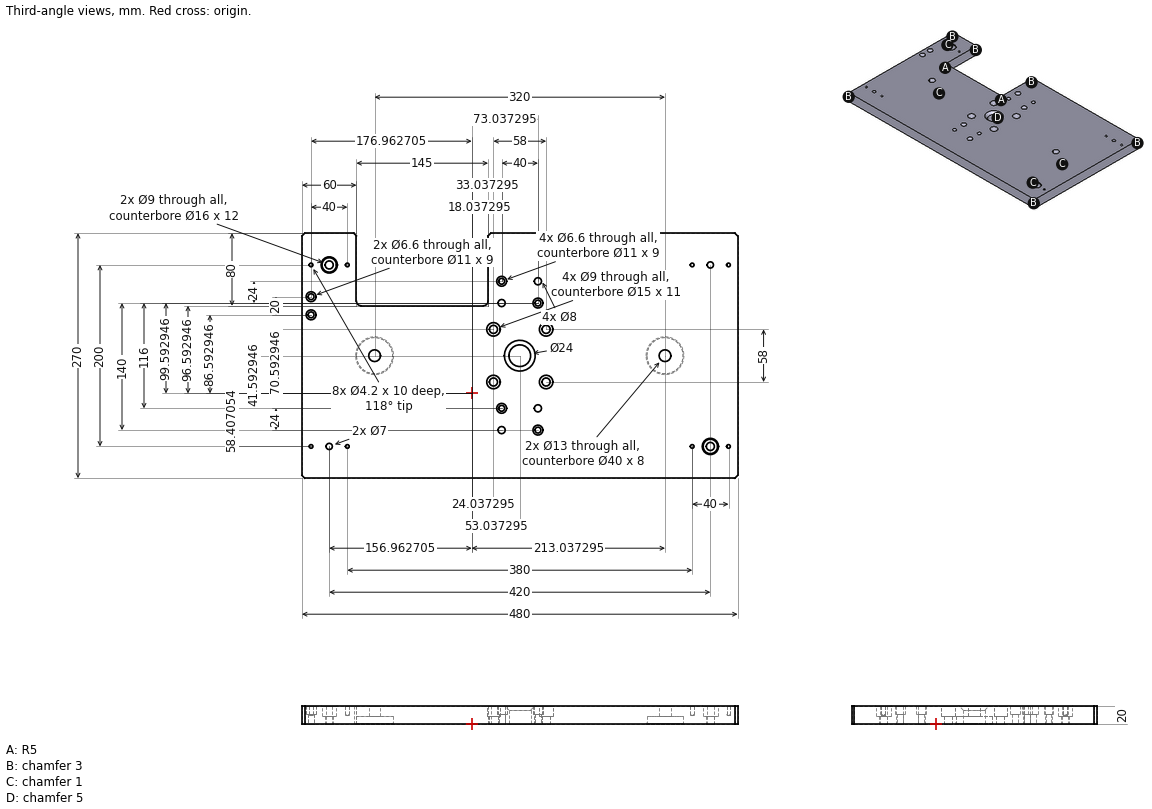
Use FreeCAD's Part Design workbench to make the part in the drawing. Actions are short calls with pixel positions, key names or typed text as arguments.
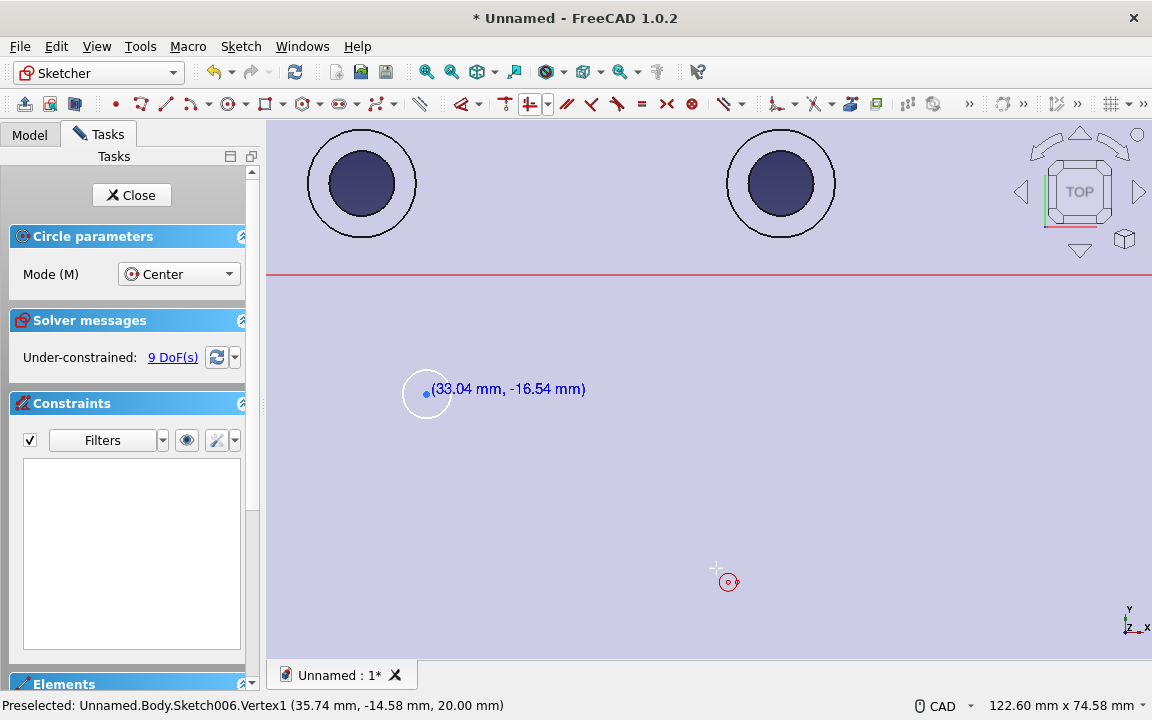
click(716, 567)
click(733, 550)
key(Escape)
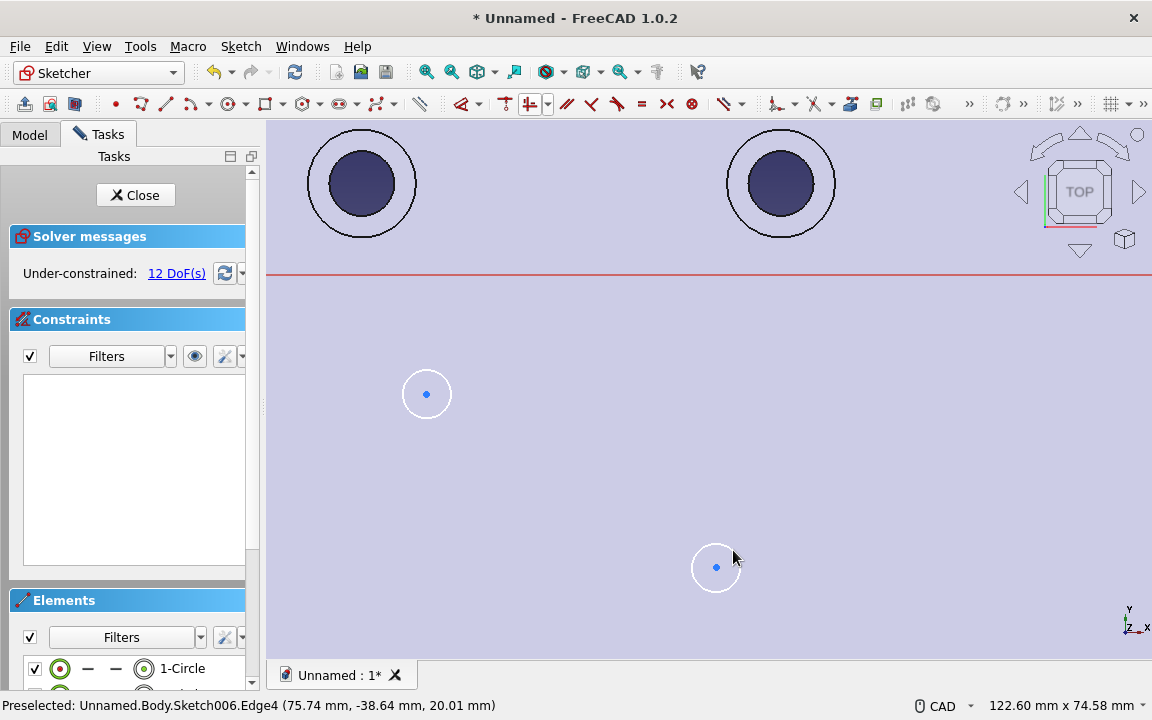
scroll(717, 569, down, 6)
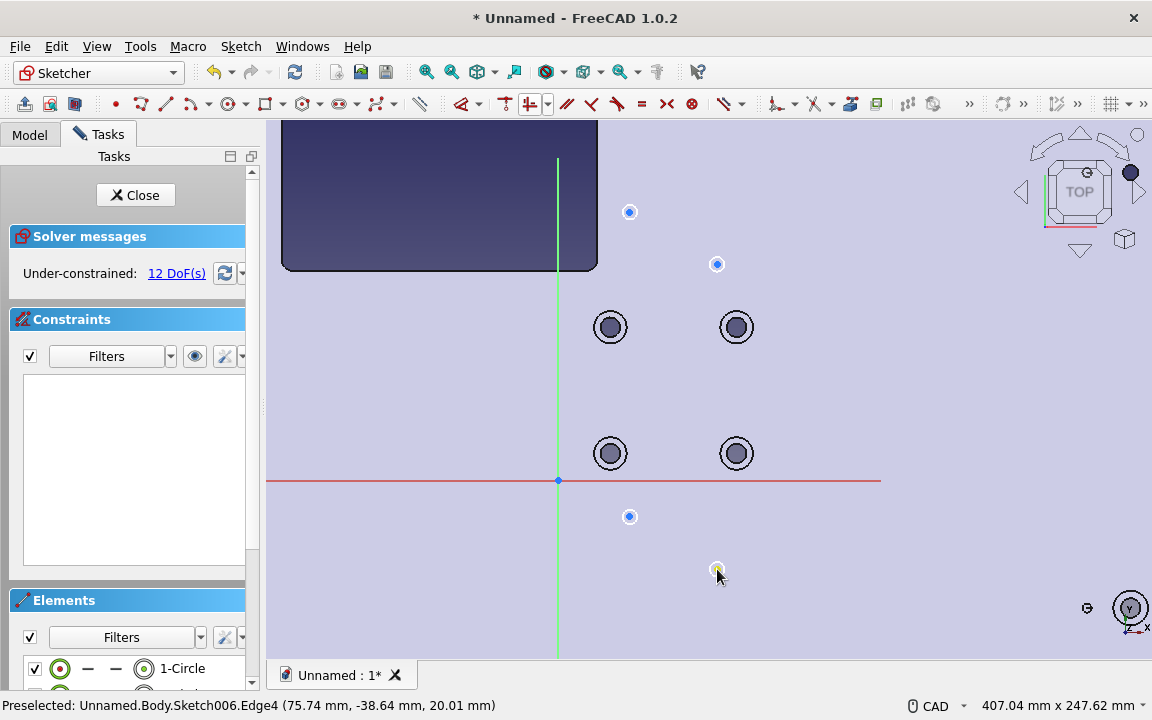
scroll(635, 207, up, 4)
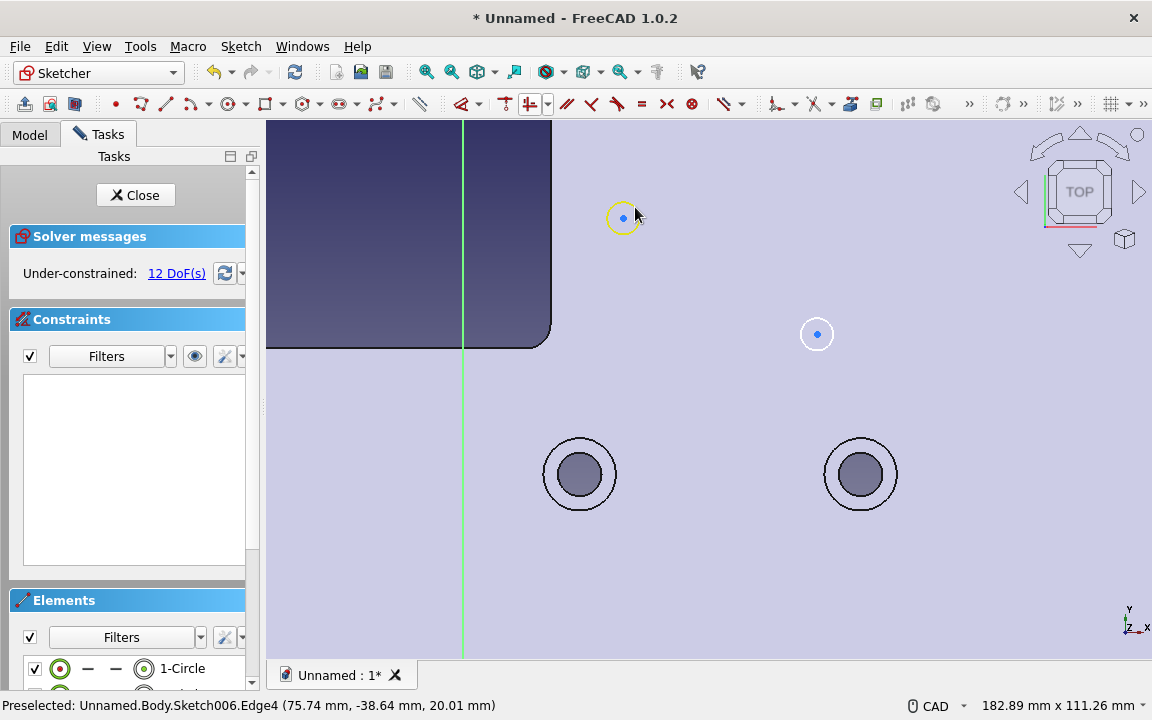
click(635, 207)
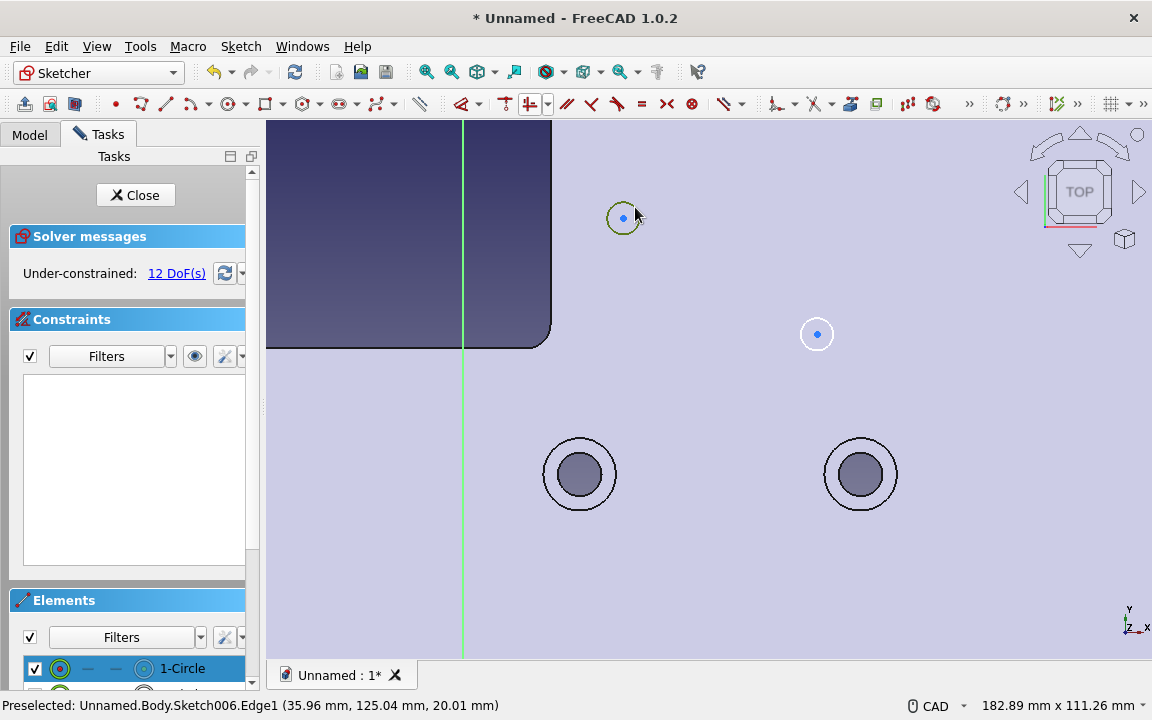
click(828, 323)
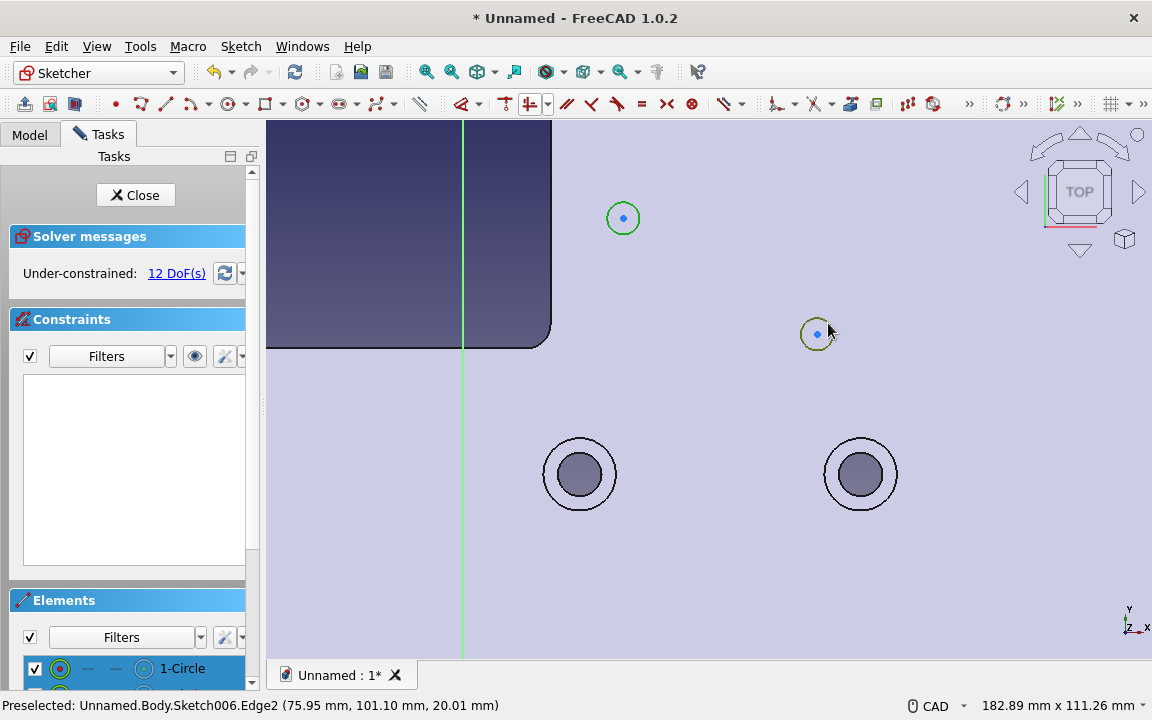
scroll(634, 206, down, 4)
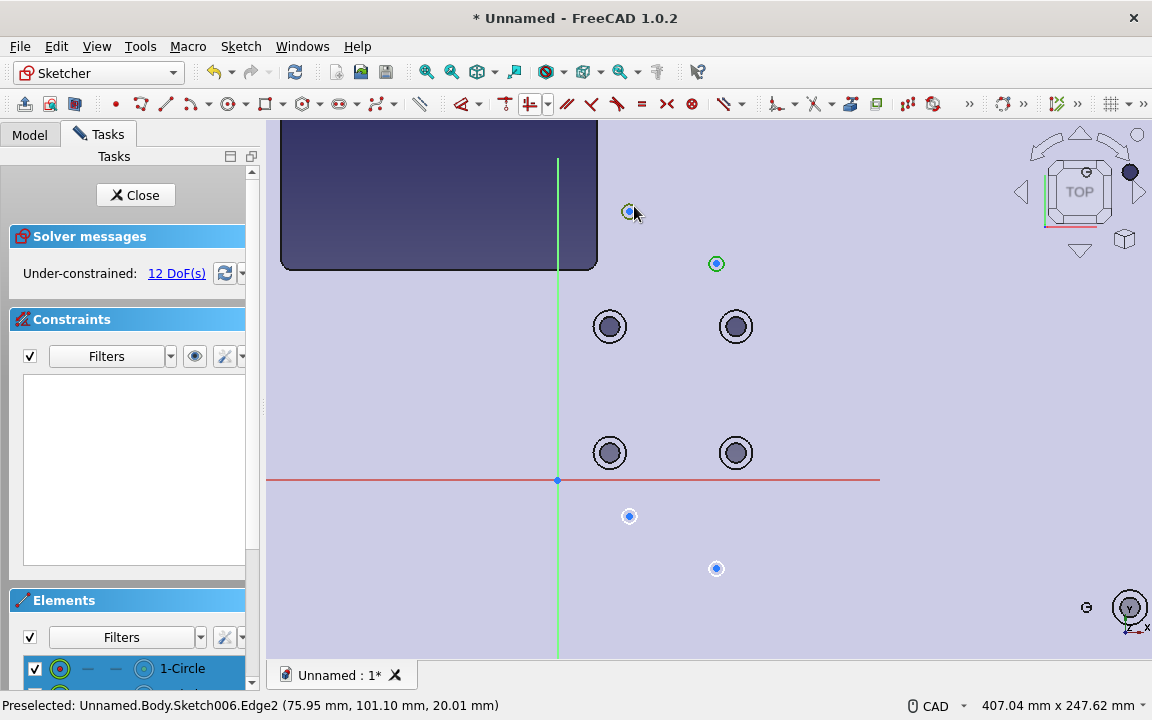
scroll(635, 511, up, 4)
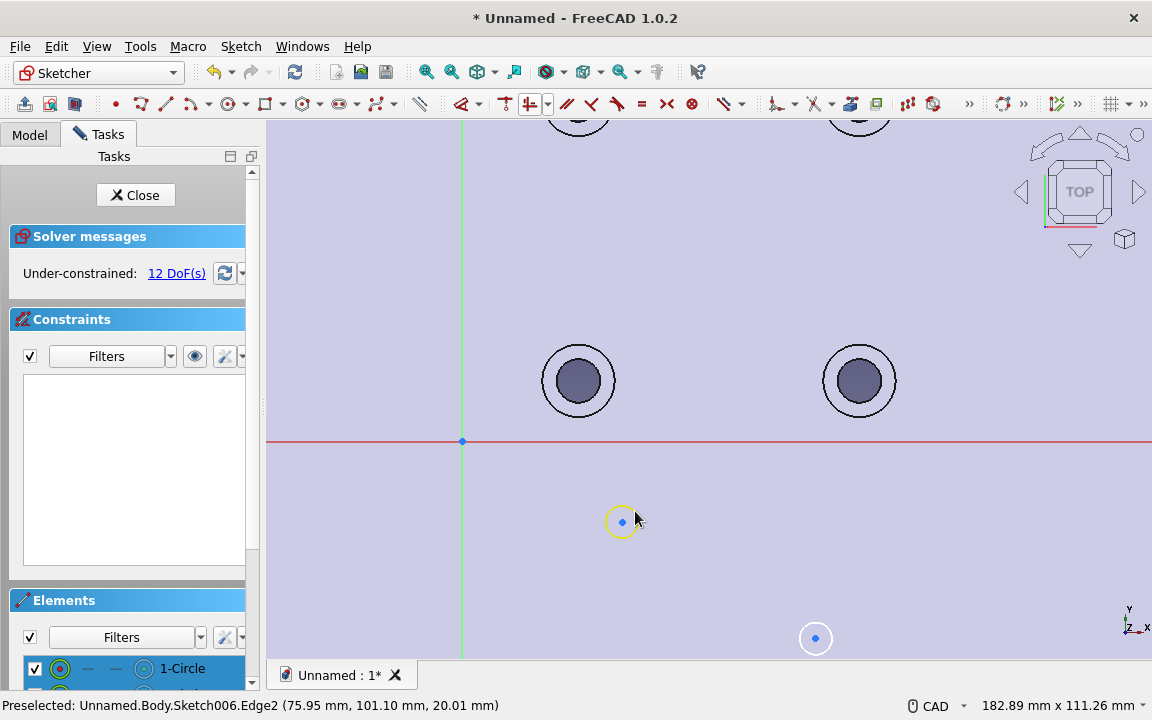
click(633, 511)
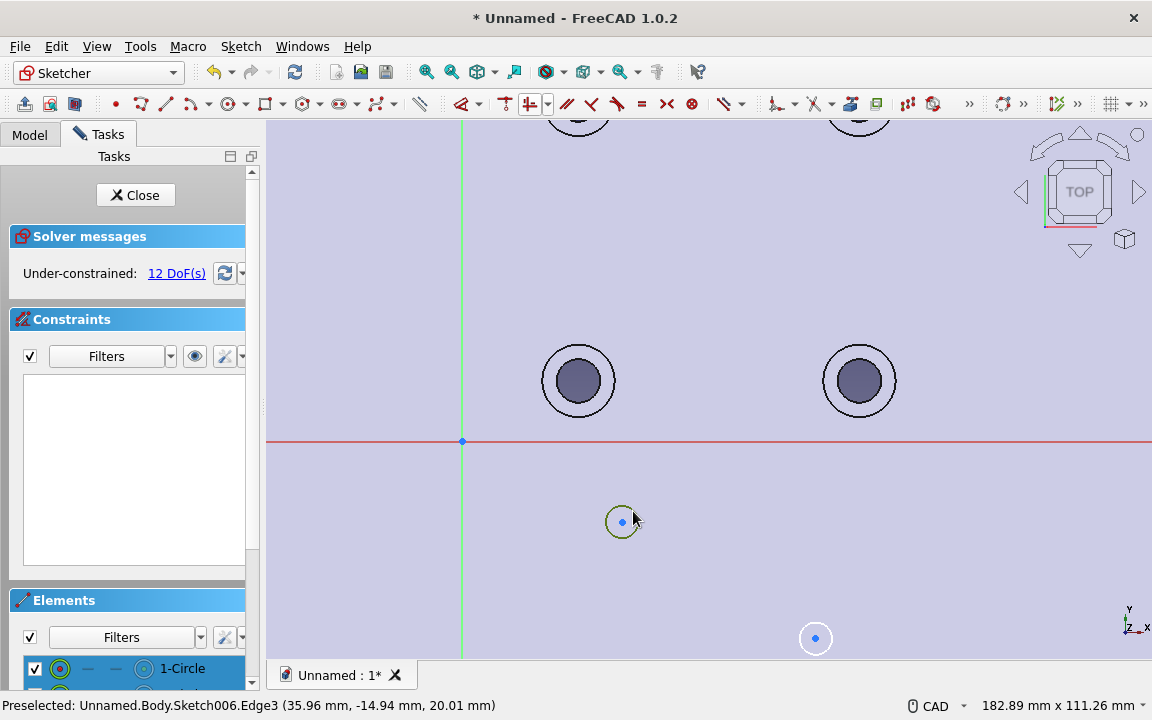
click(827, 627)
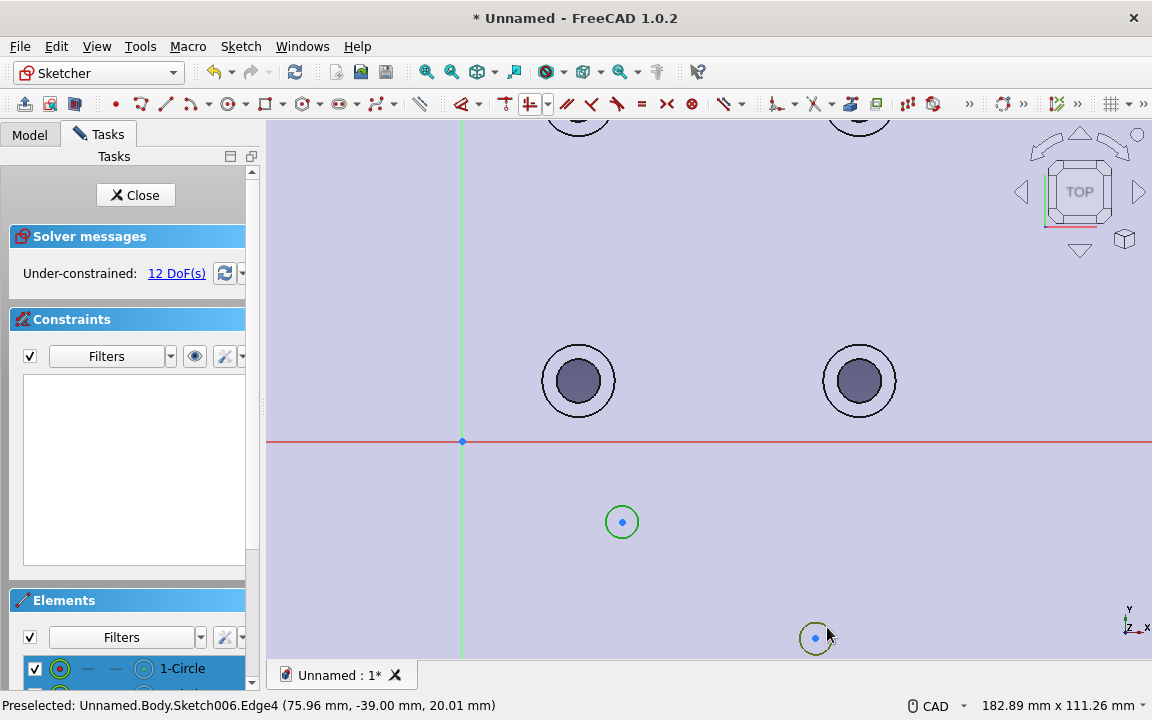
key(e)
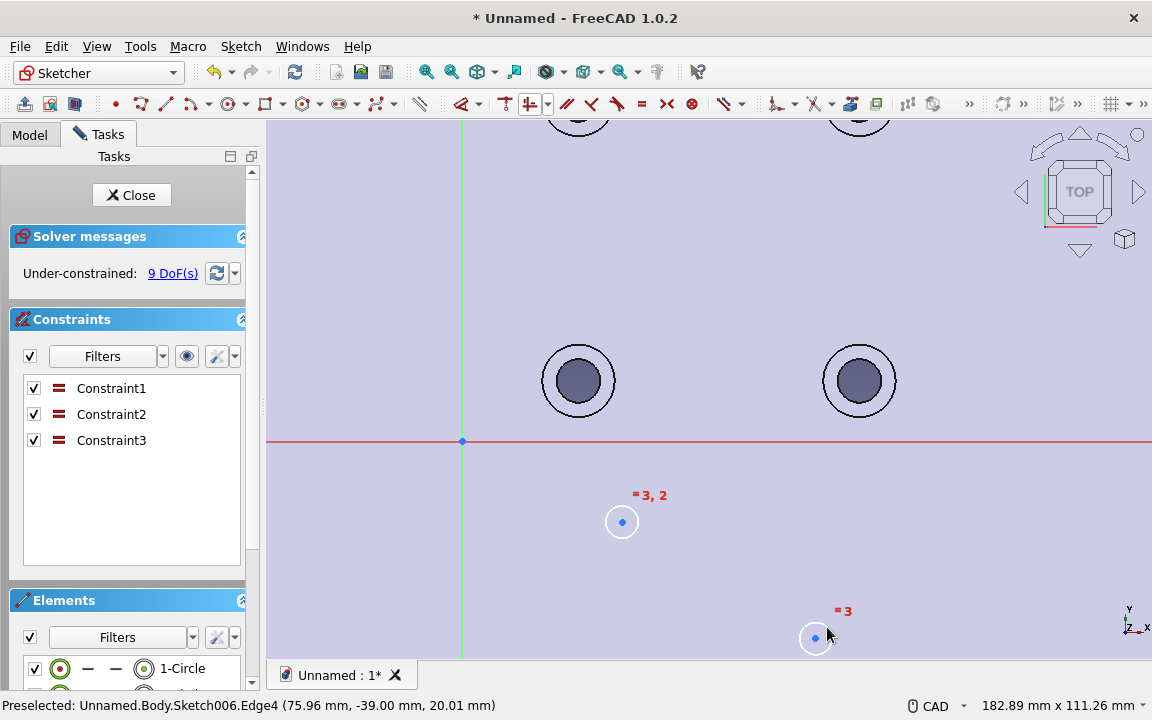
scroll(635, 511, down, 4)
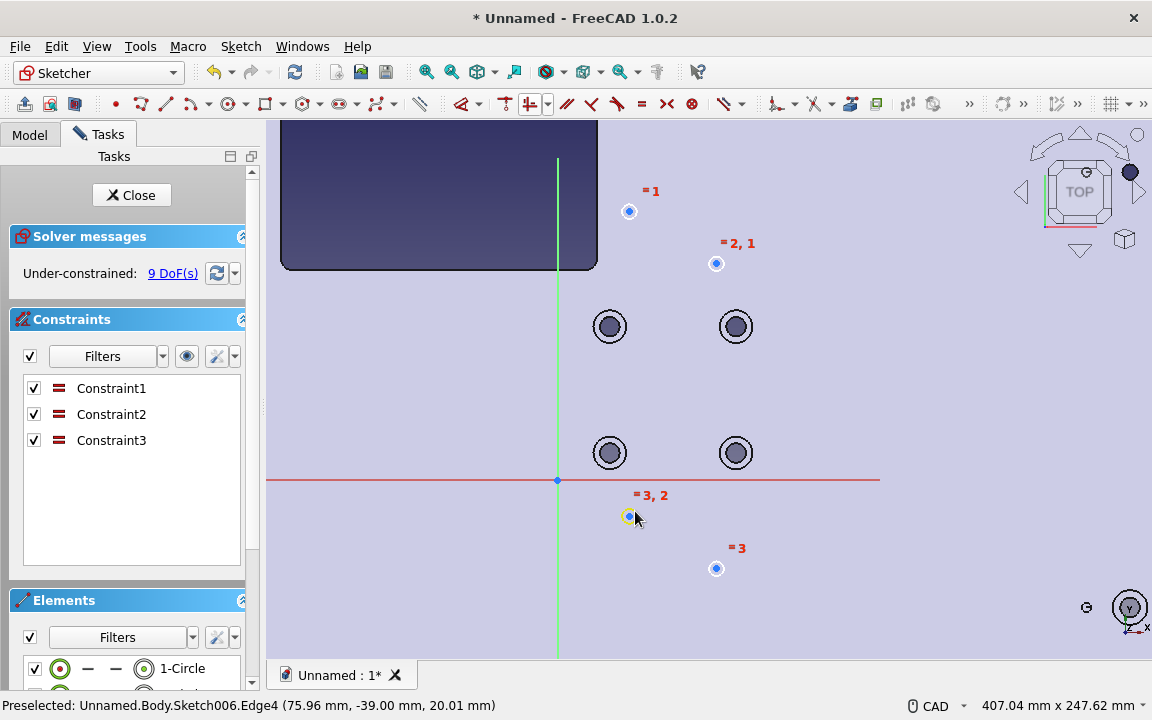
click(629, 212)